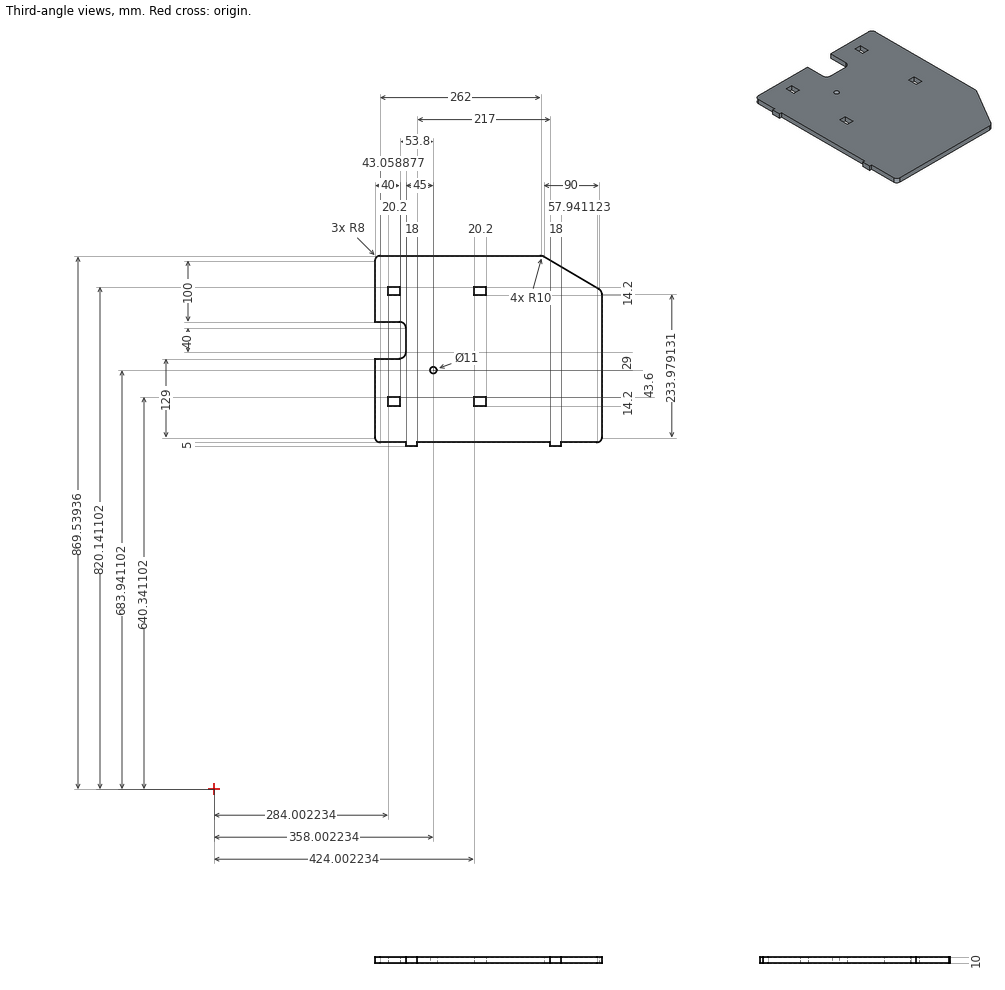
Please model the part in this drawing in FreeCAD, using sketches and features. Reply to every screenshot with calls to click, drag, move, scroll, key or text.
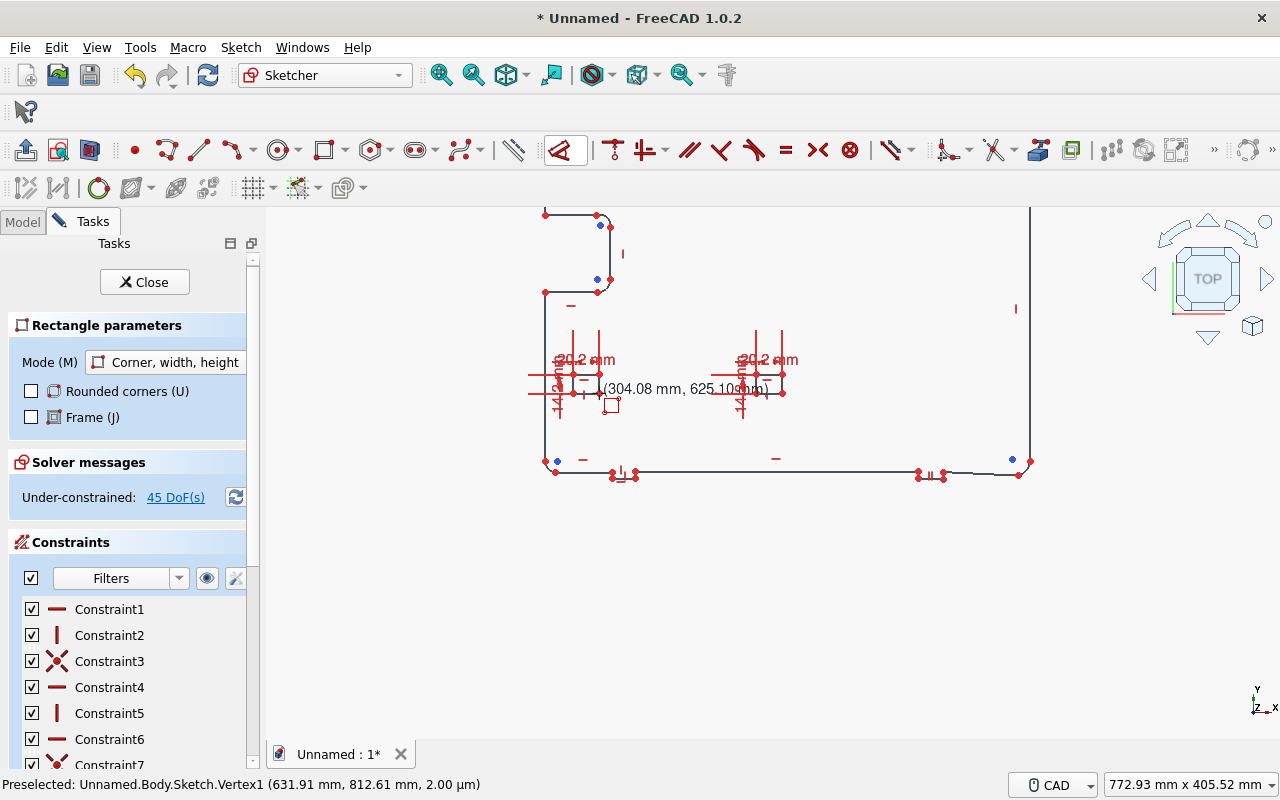
scroll(743, 400, down, 6)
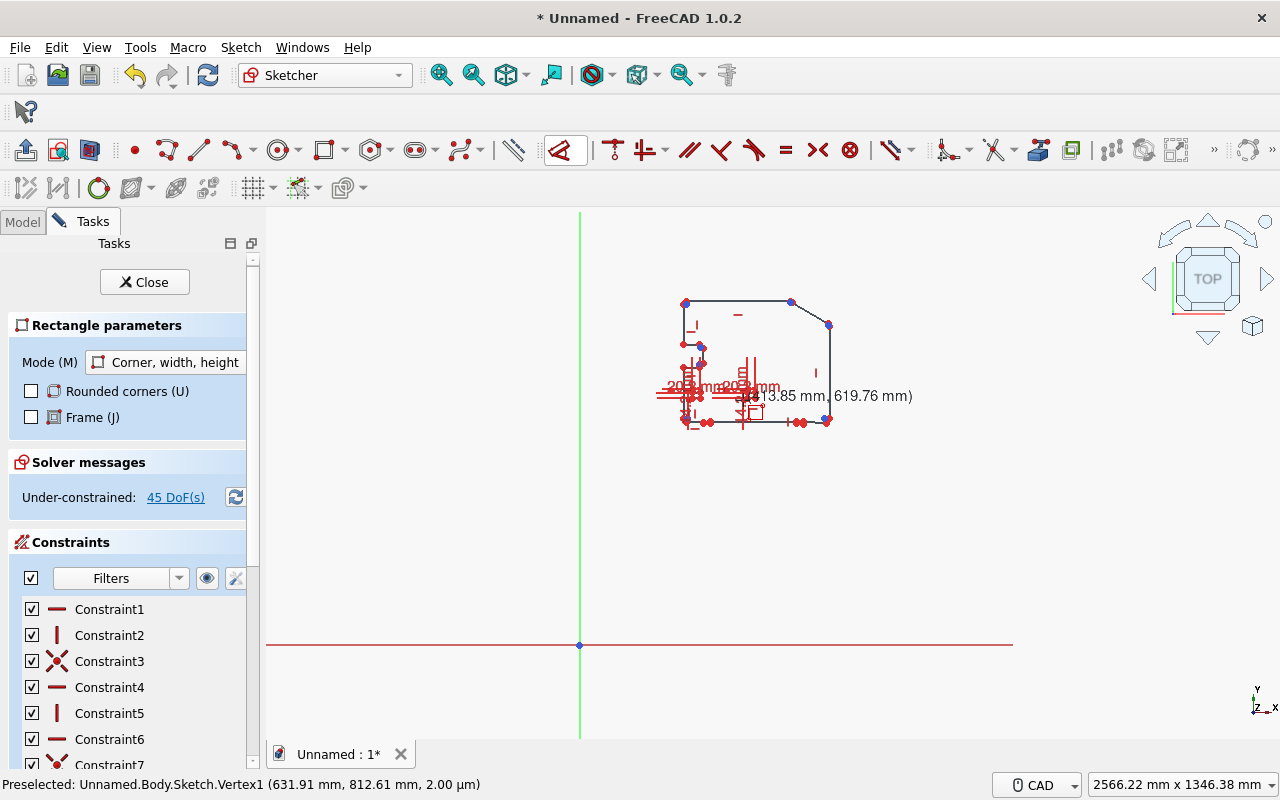
scroll(747, 321, up, 6)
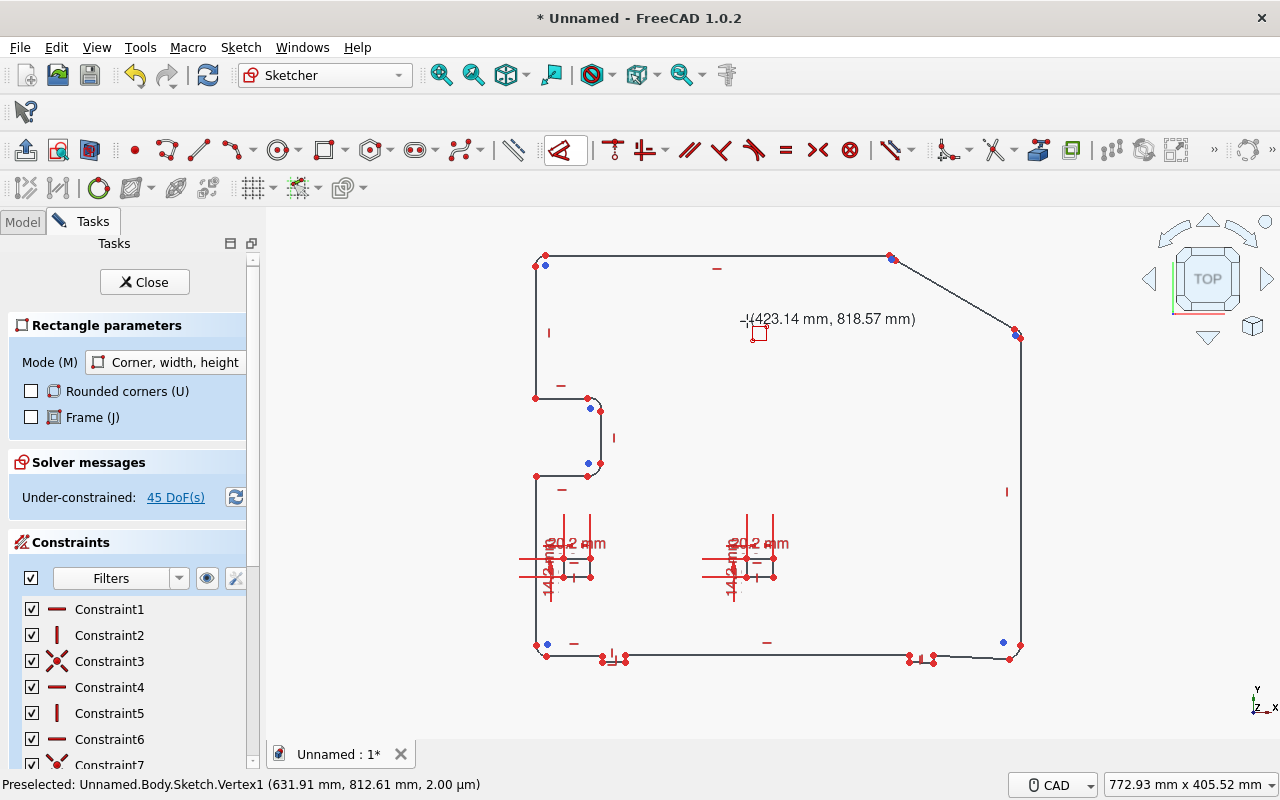
click(747, 322)
move(774, 340)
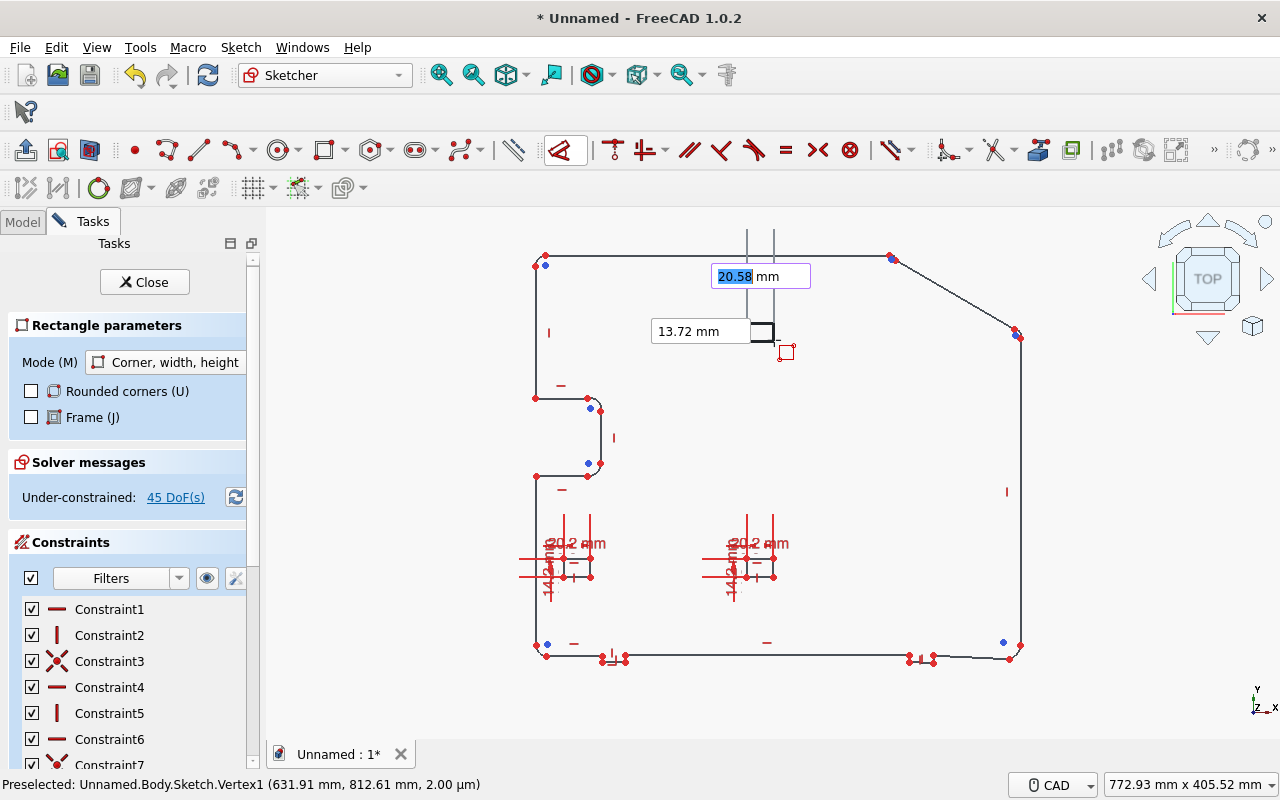
text(20.2)
key(Tab)
text(14.2)
key(Return)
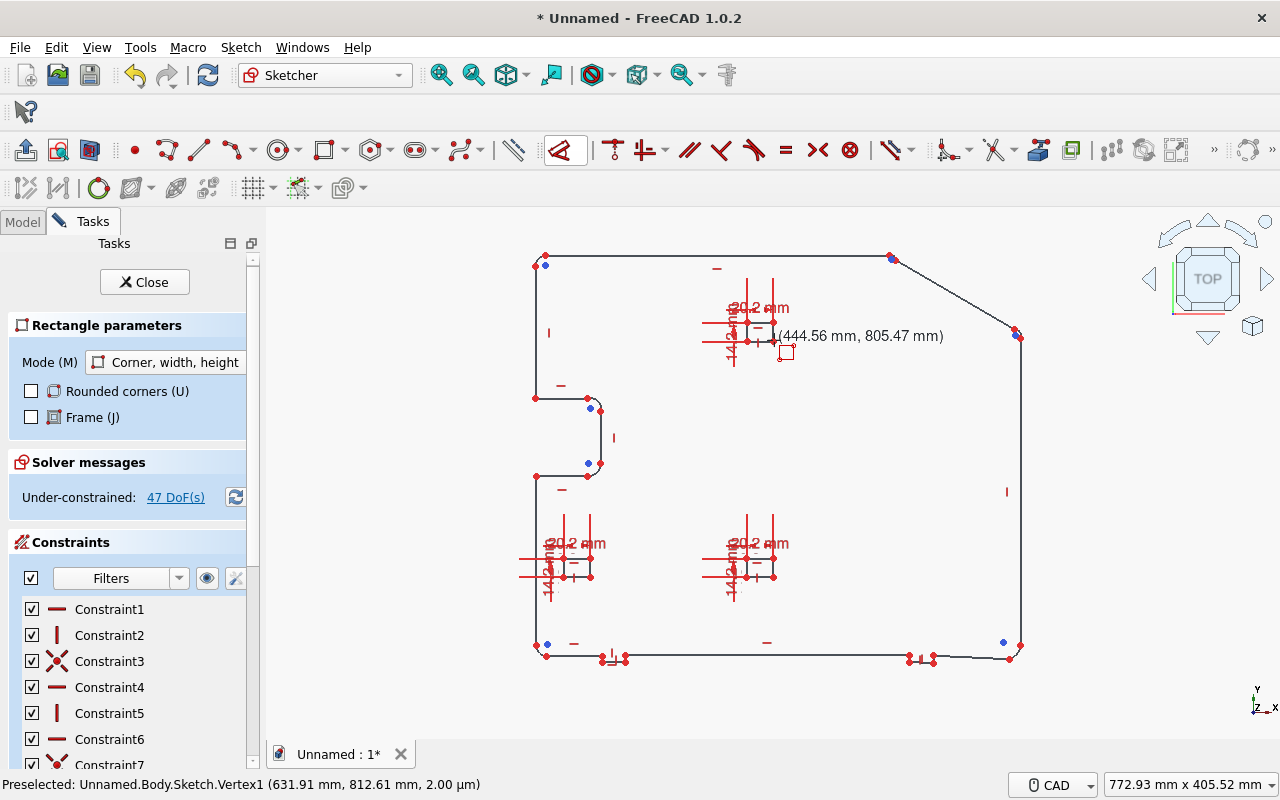
click(563, 322)
move(590, 340)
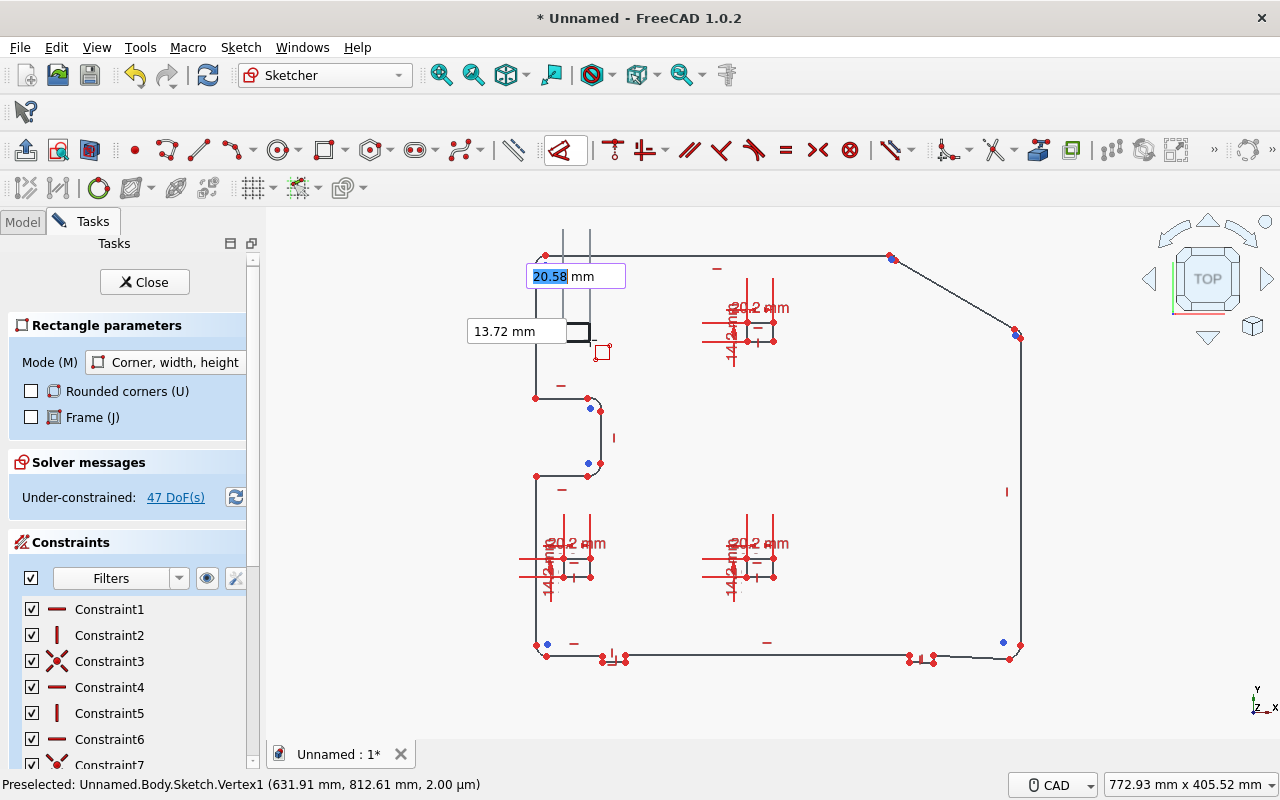
text(20.2)
key(Tab)
text(14.2)
key(Return)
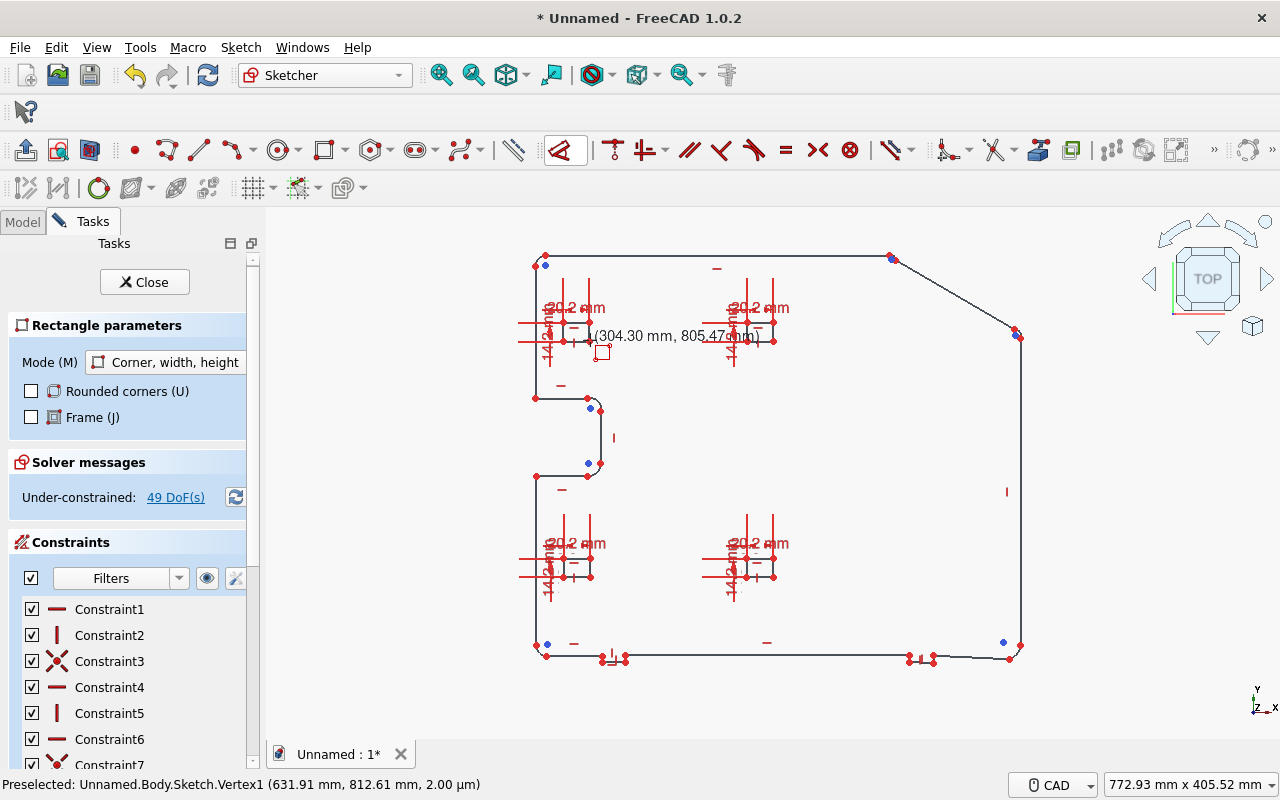
click(278, 150)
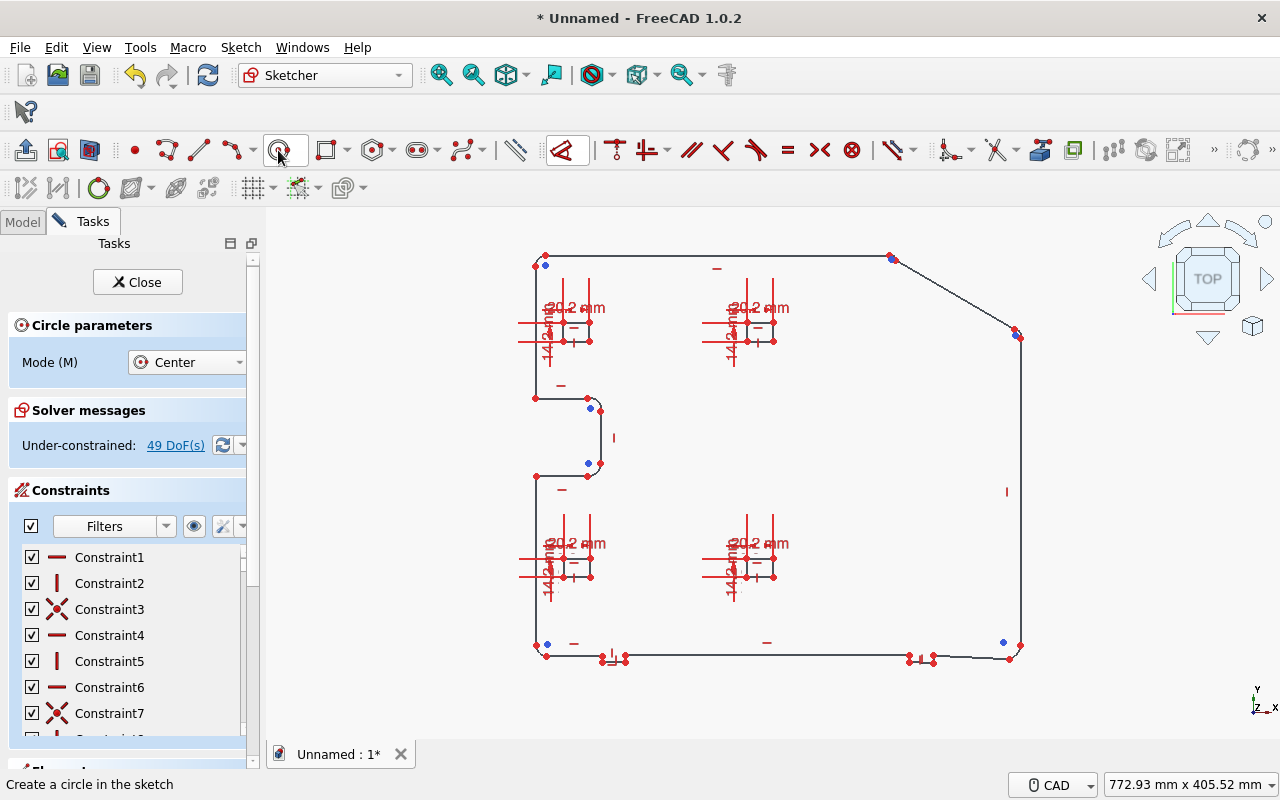
scroll(660, 500, up, 6)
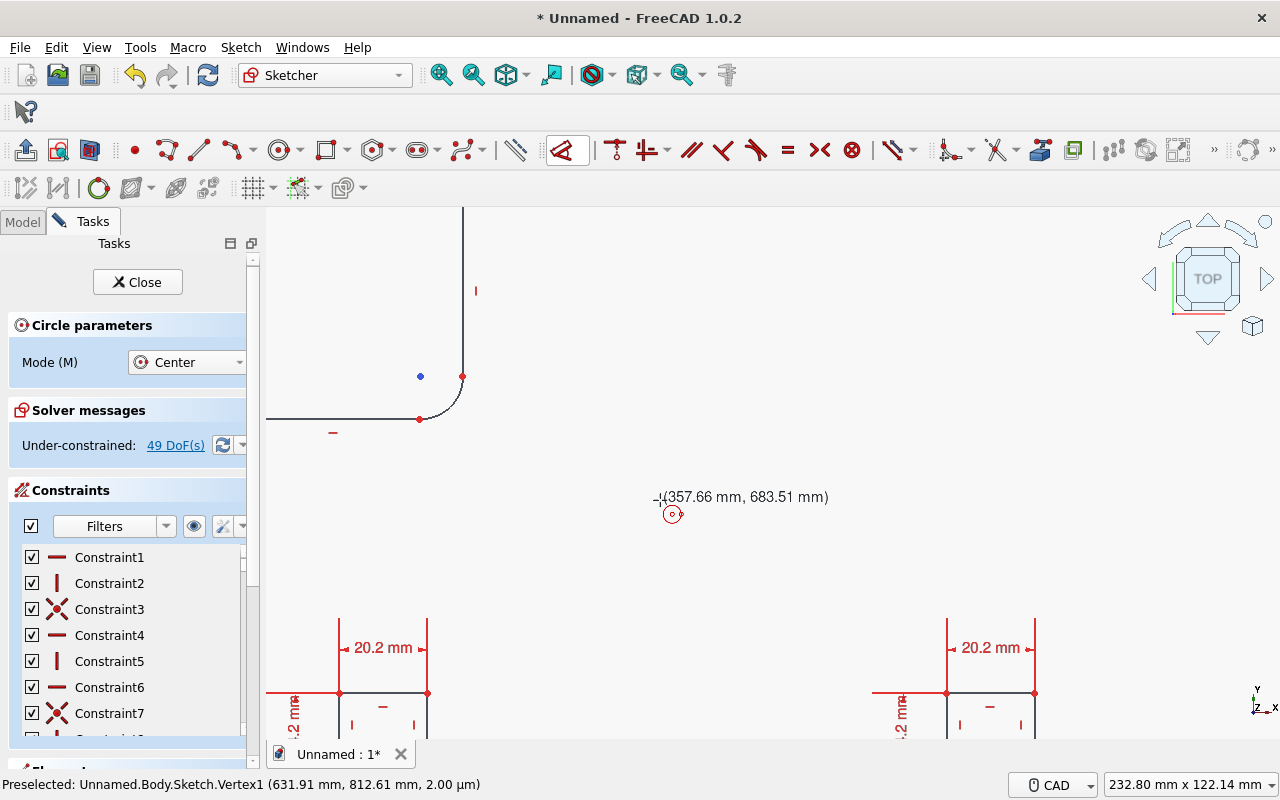
scroll(727, 362, down, 12)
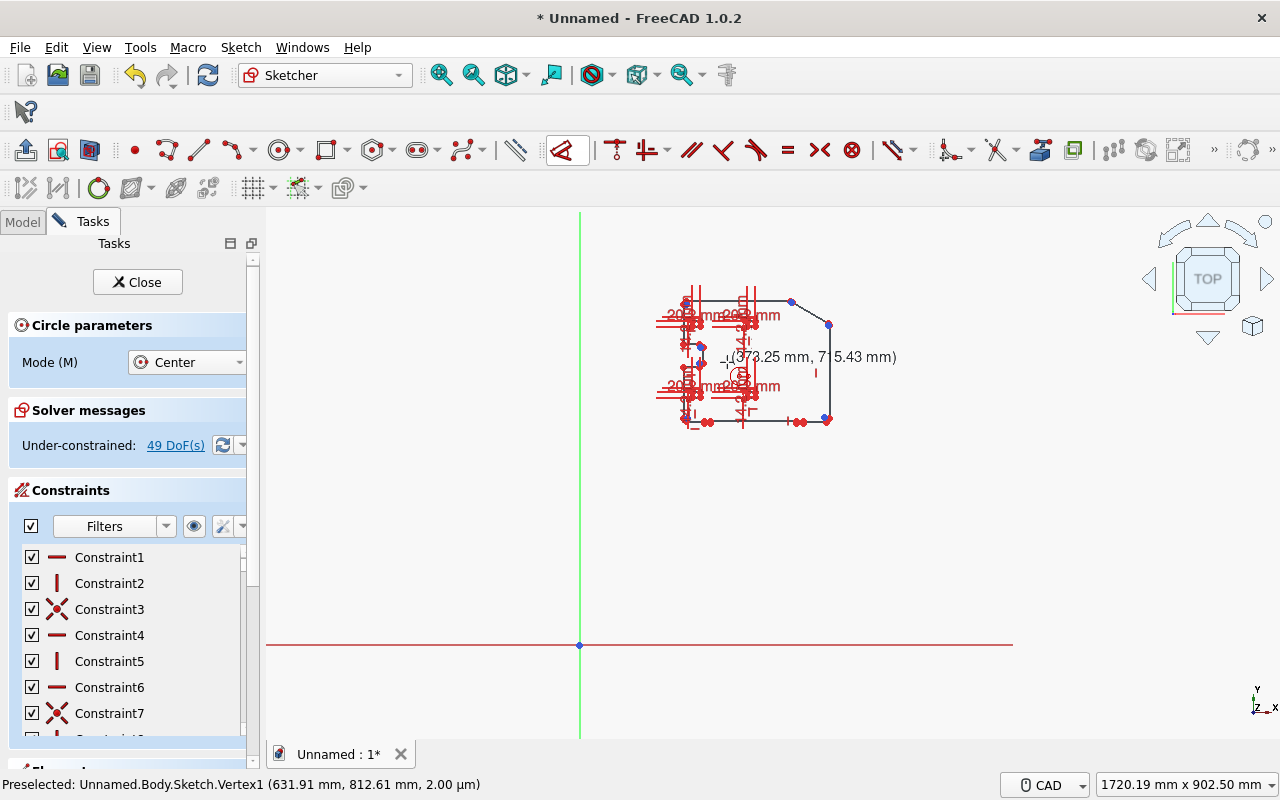
click(721, 375)
move(723, 373)